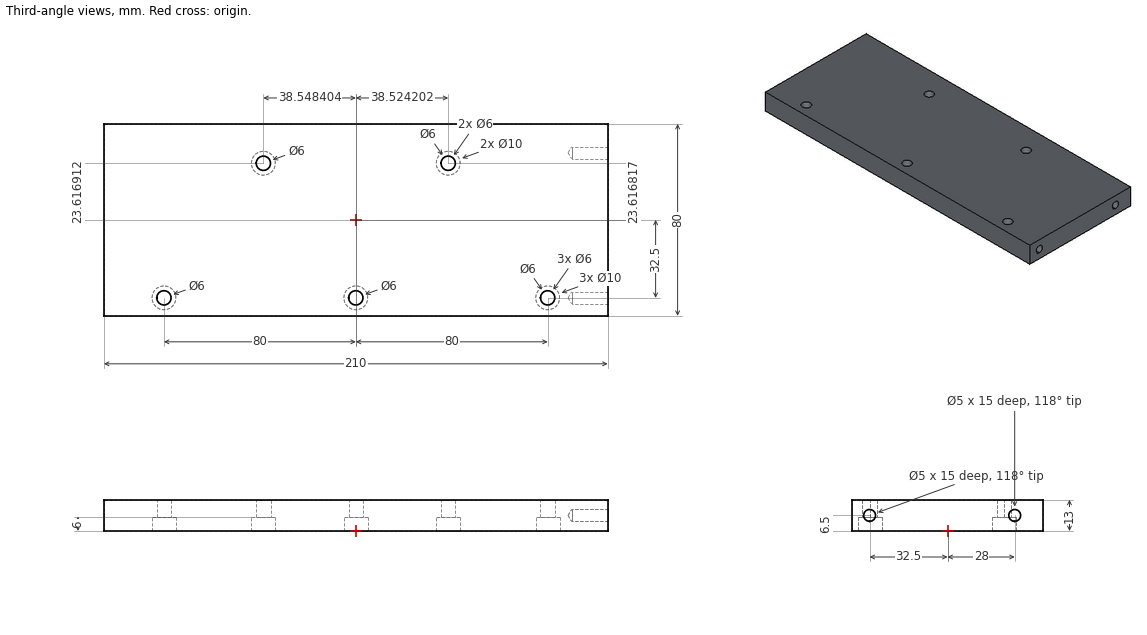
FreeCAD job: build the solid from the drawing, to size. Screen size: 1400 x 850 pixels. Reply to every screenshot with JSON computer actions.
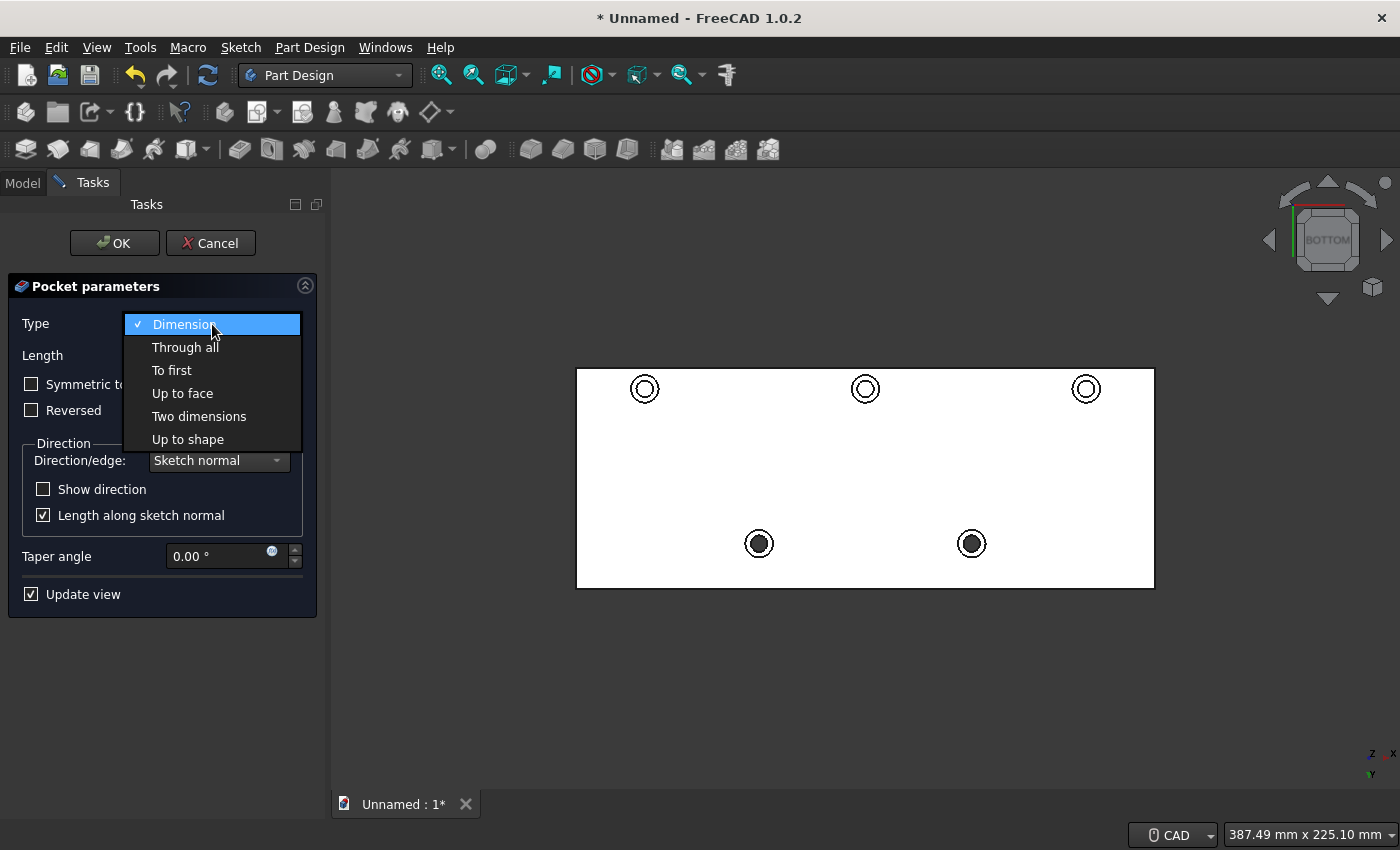
{"action": "left_click", "coordinate": [212, 370]}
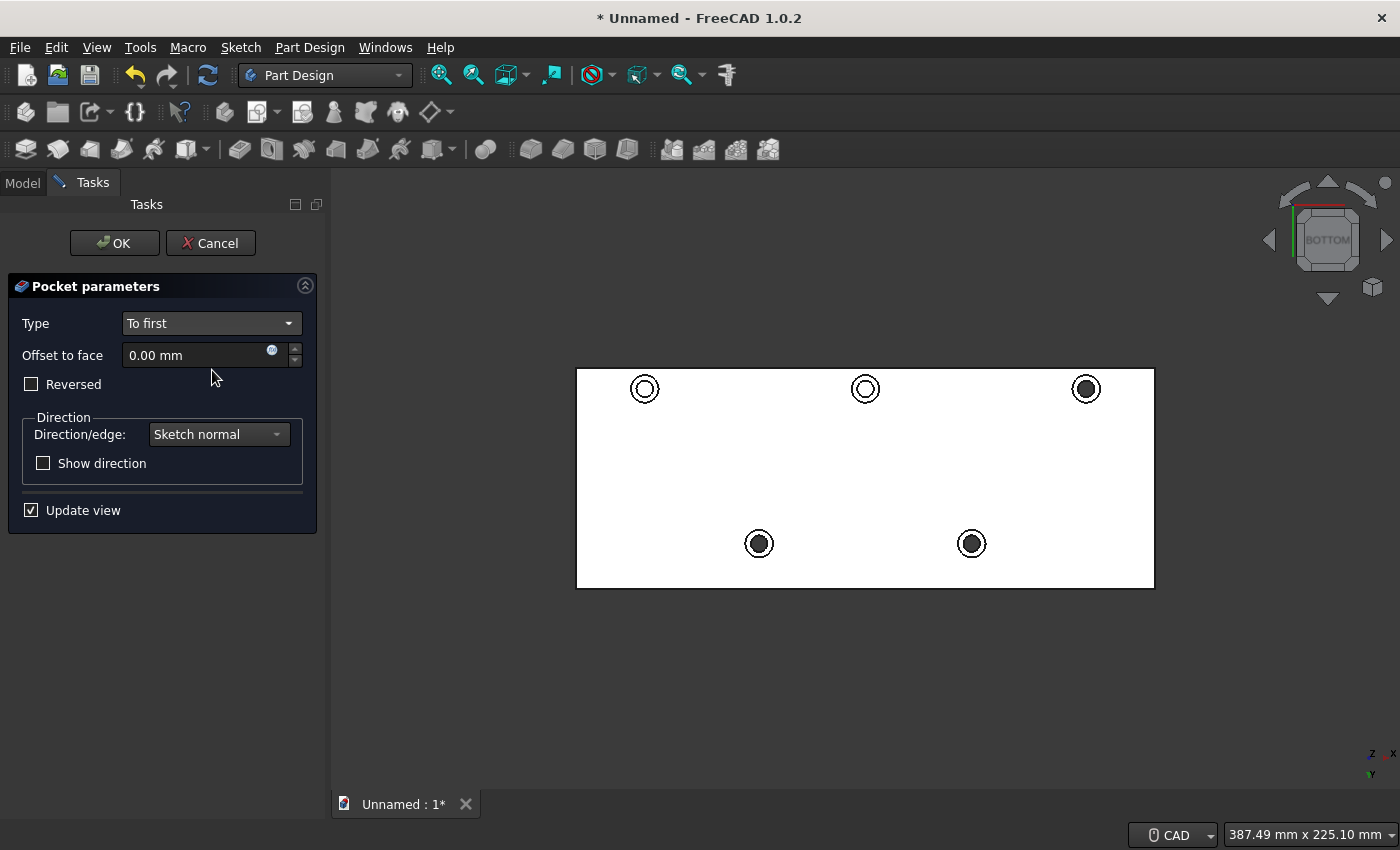
{"action": "left_click", "coordinate": [115, 243]}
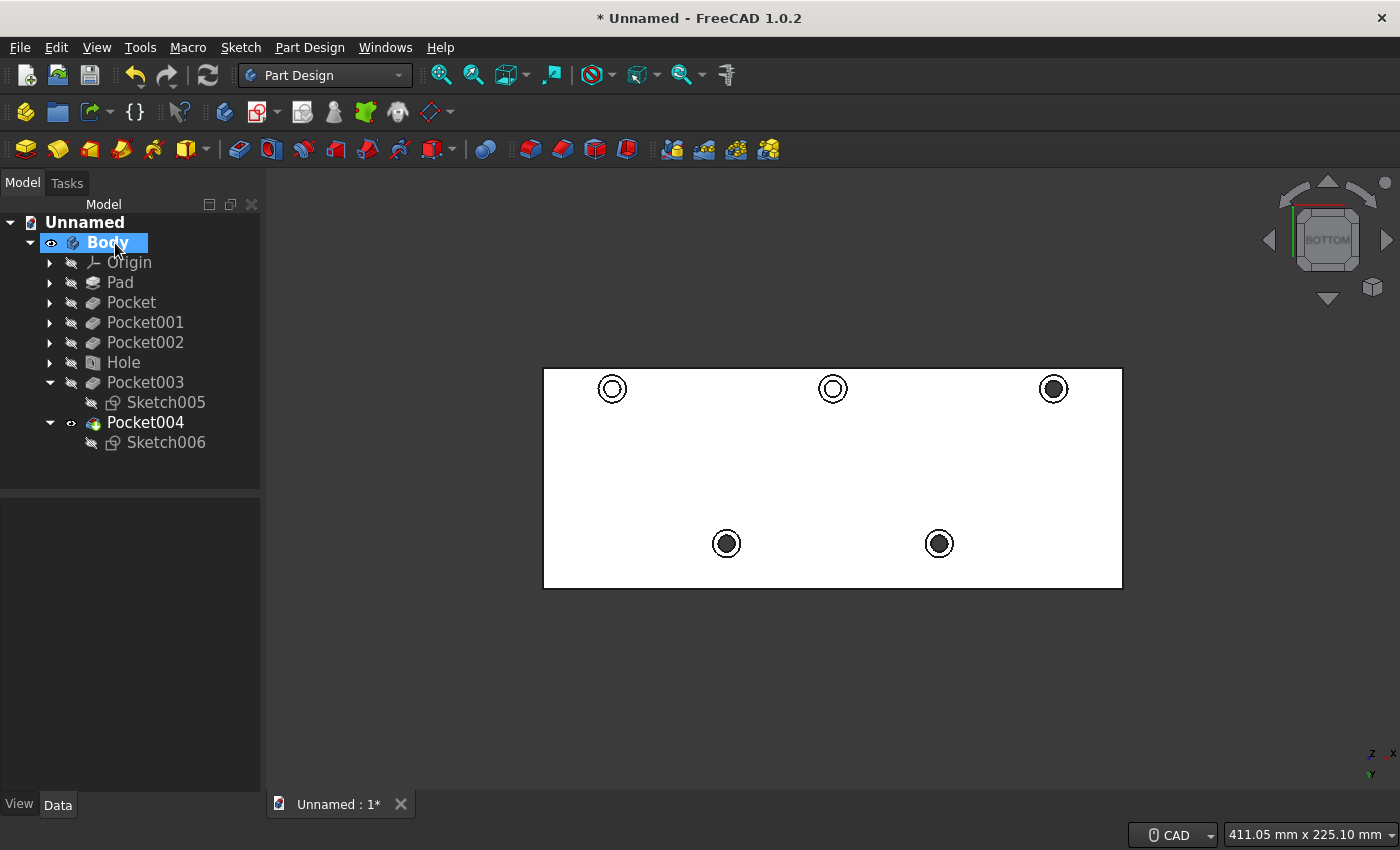
{"action": "left_click", "coordinate": [258, 112]}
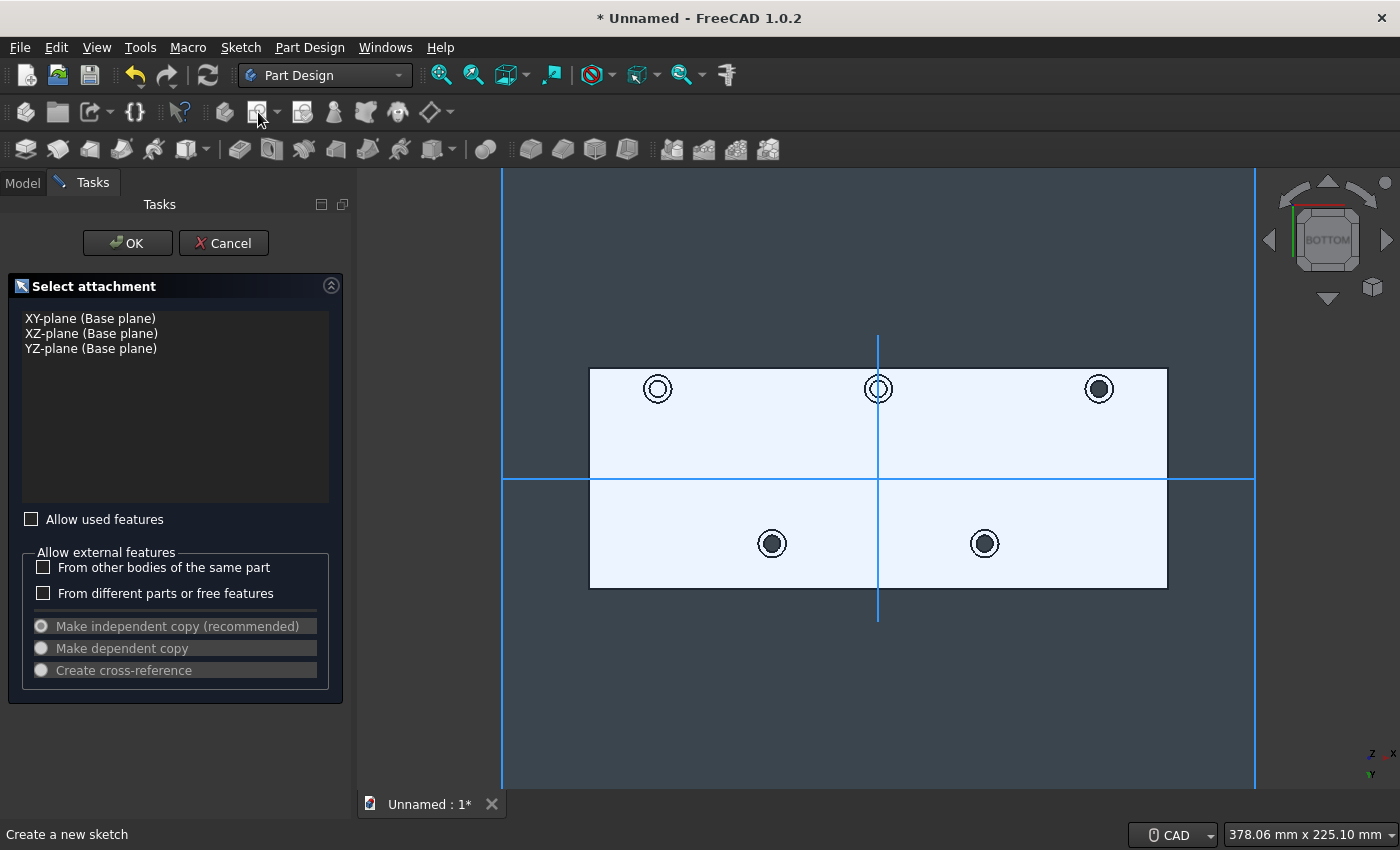
{"action": "left_click", "coordinate": [82, 318]}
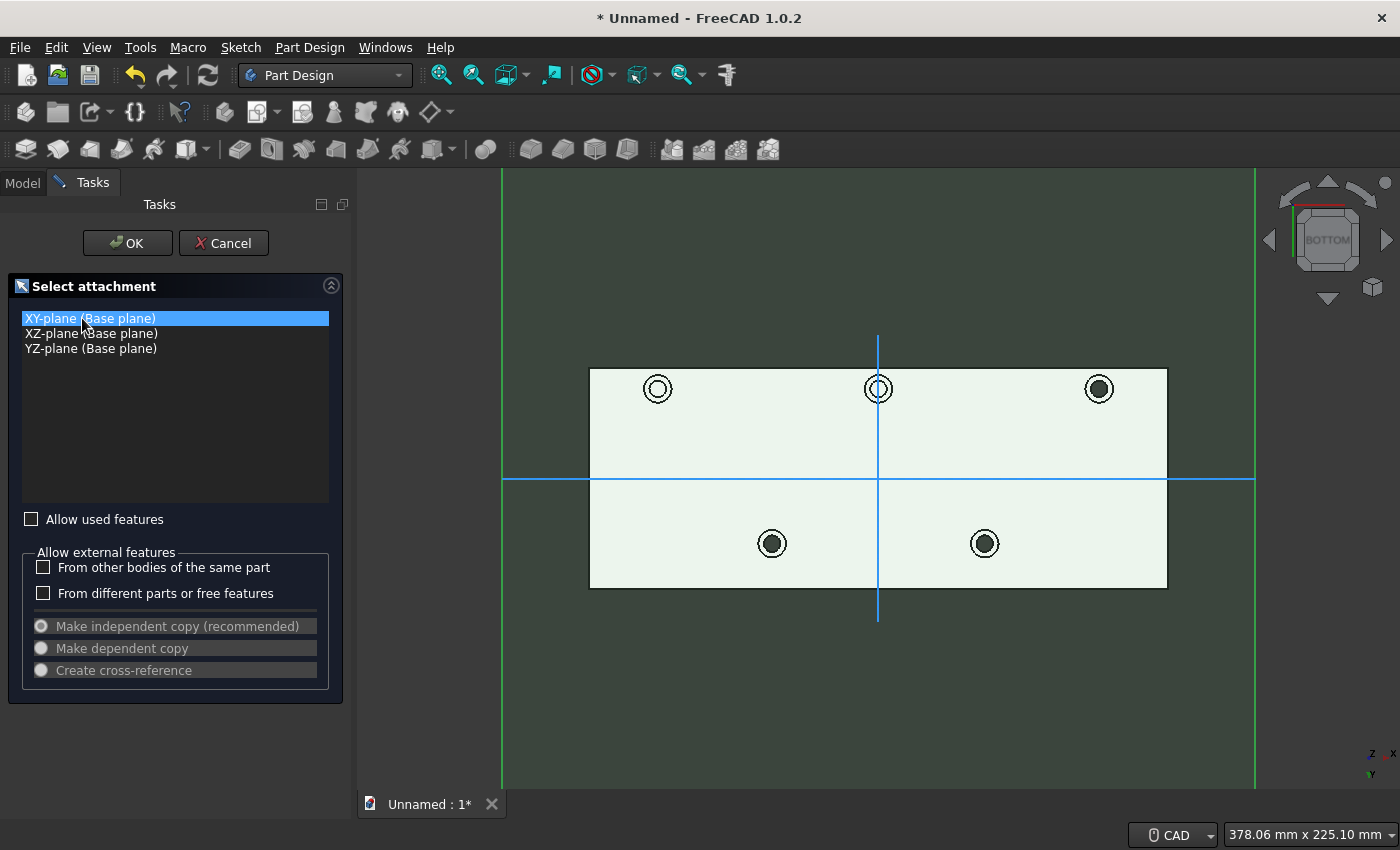
{"action": "left_click", "coordinate": [128, 243]}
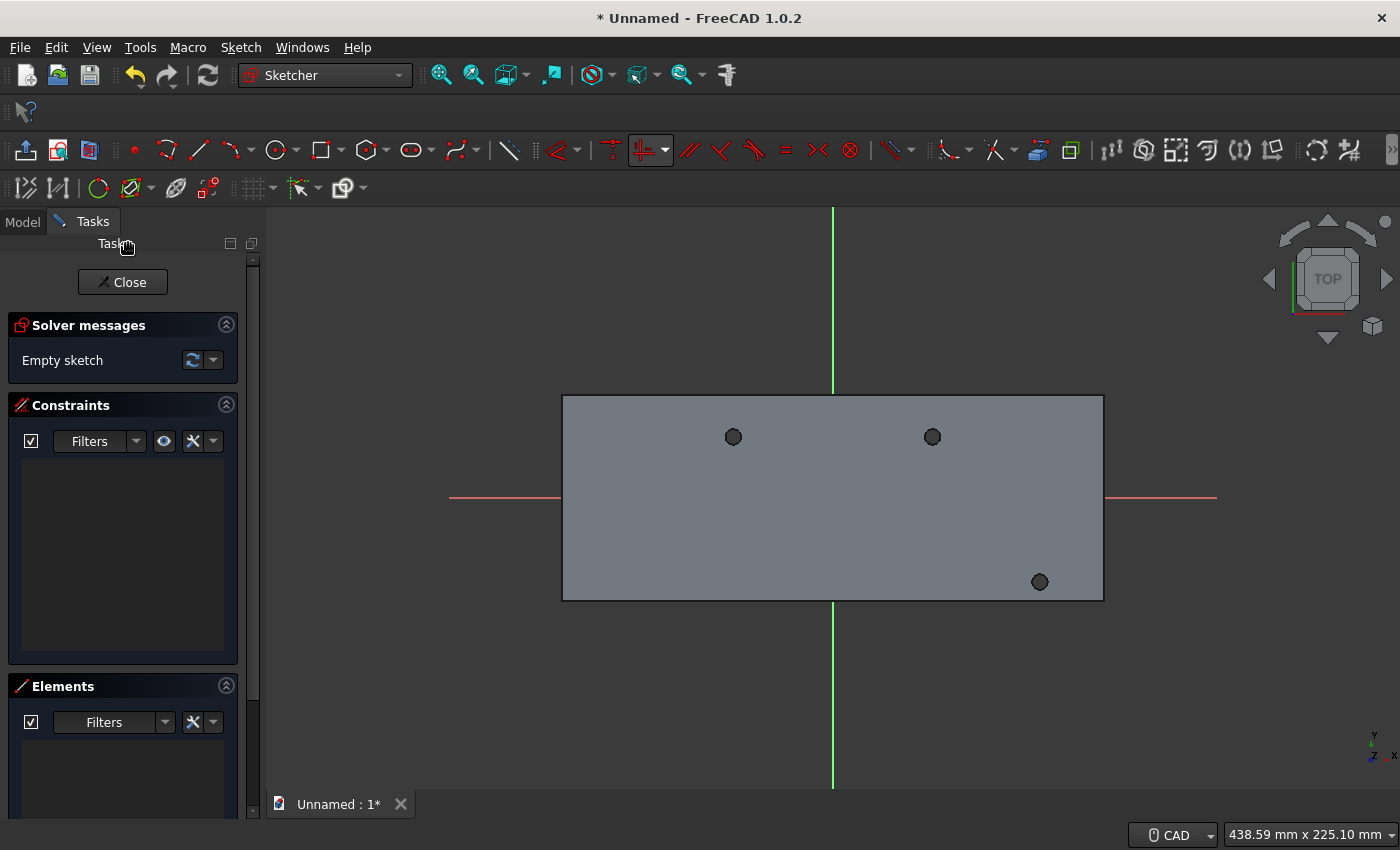
{"action": "key", "text": "q s"}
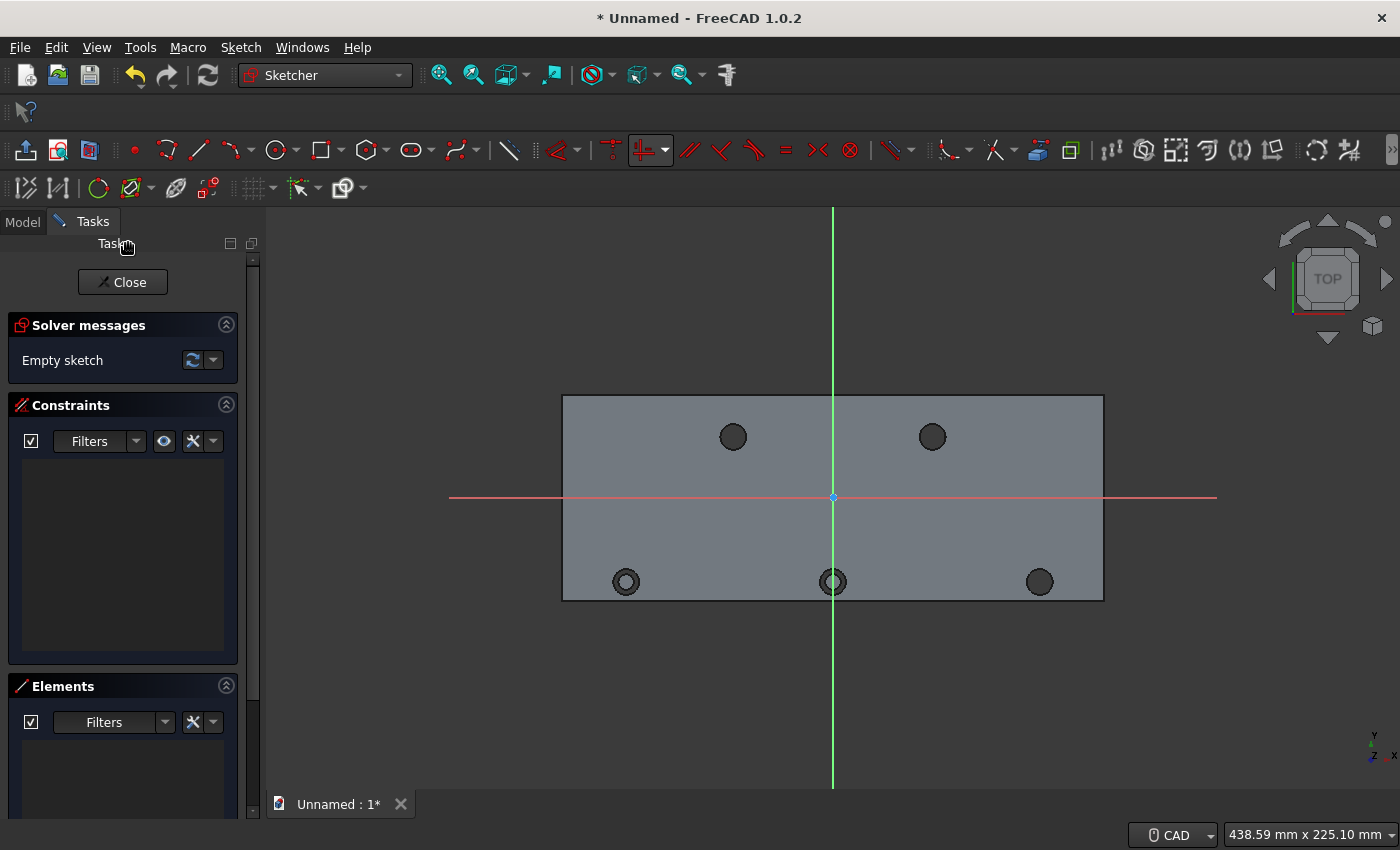
{"action": "scroll", "coordinate": [837, 586], "scroll_direction": "up", "scroll_amount": 15}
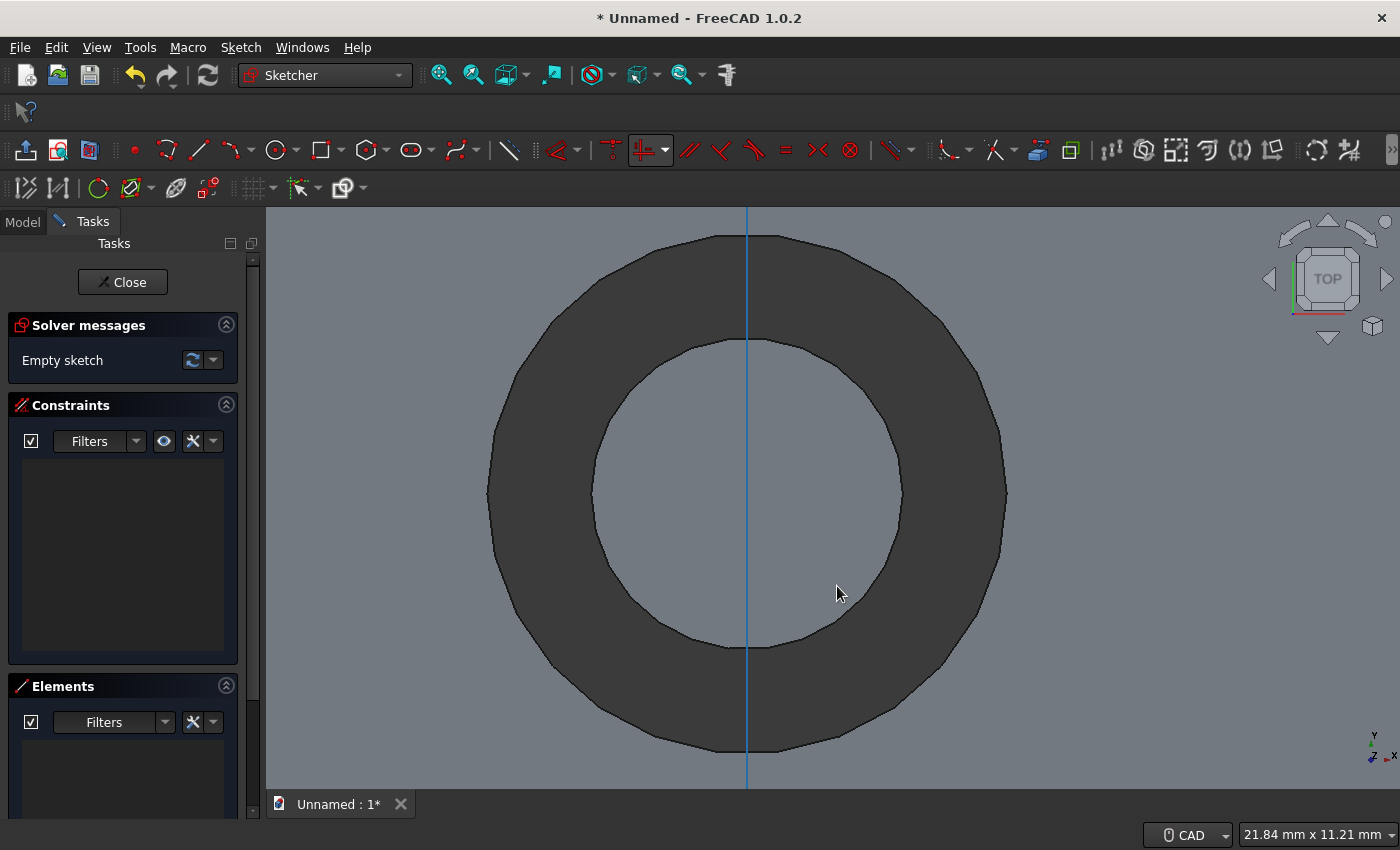
{"action": "left_click", "coordinate": [276, 150]}